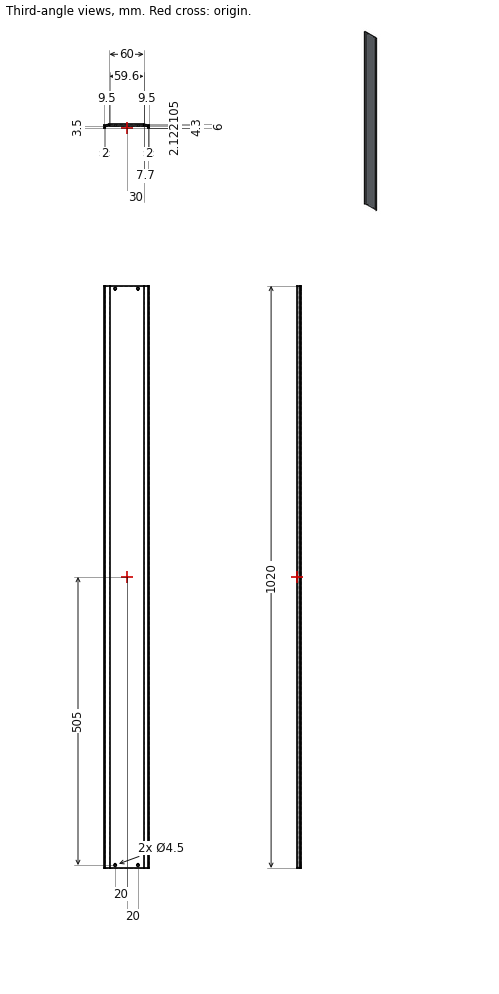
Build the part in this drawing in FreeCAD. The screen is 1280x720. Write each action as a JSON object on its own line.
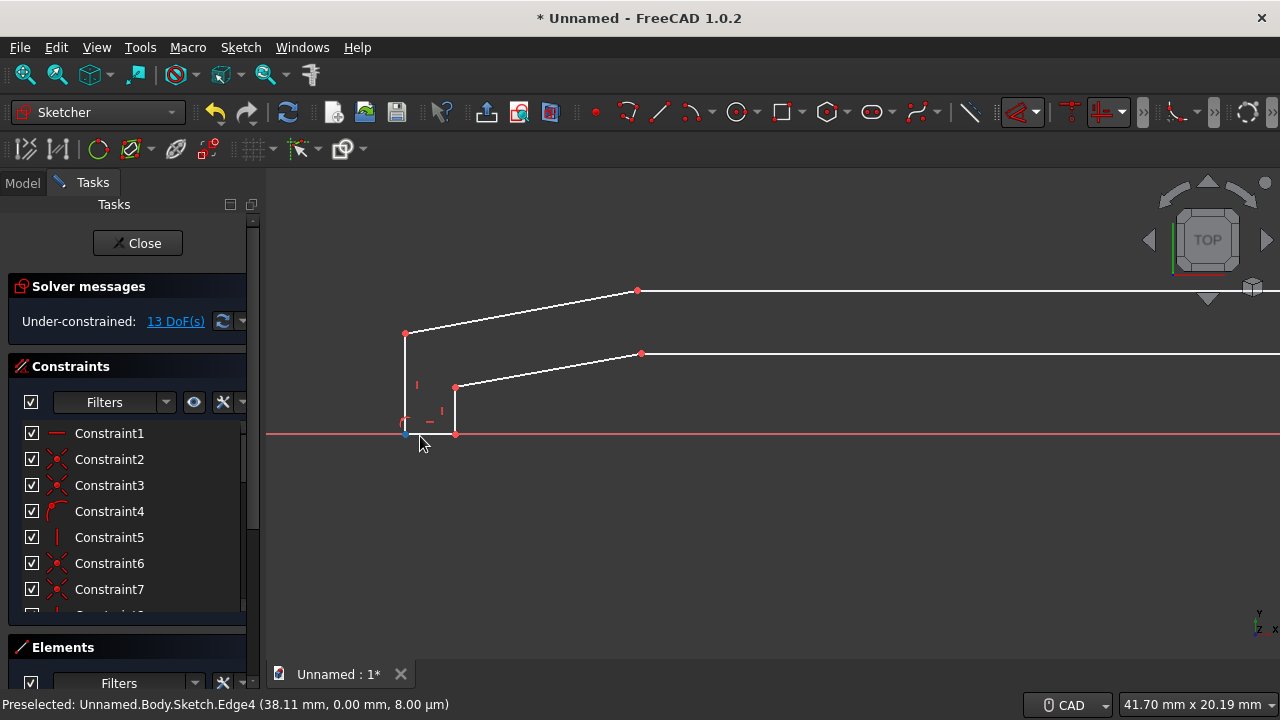
{"action": "left_click", "coordinate": [420, 434]}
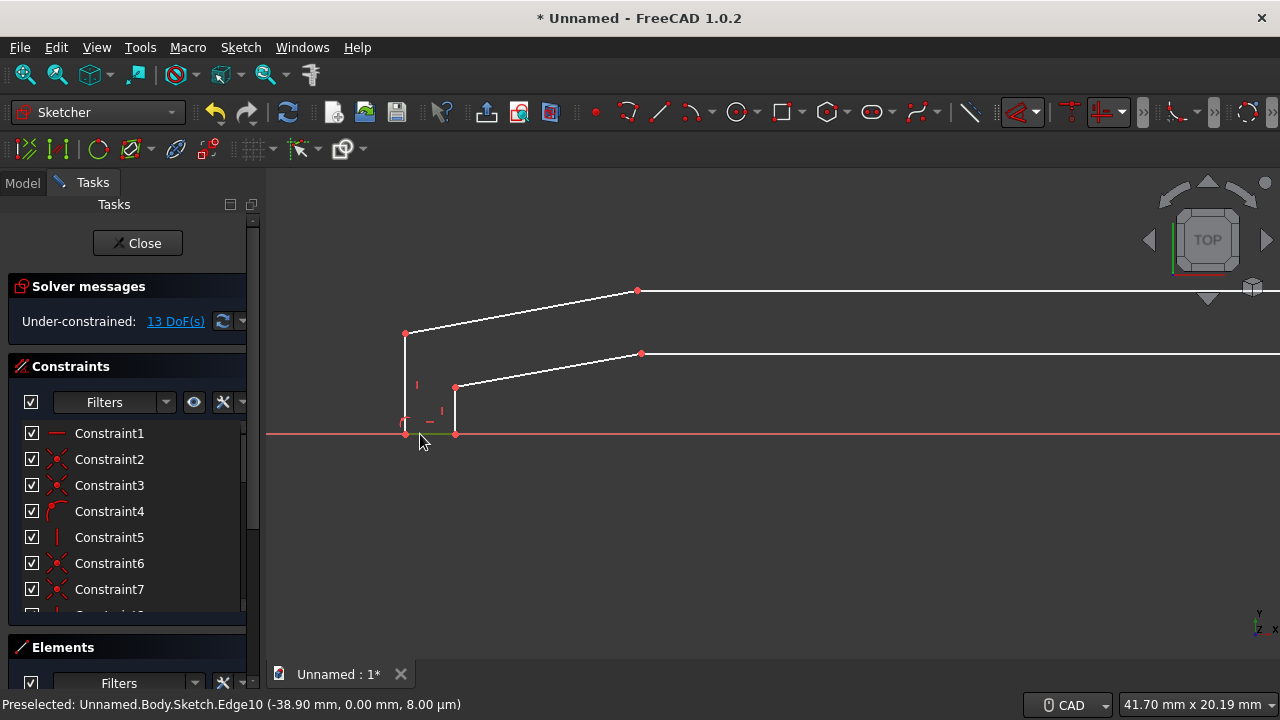
{"action": "key", "text": "l"}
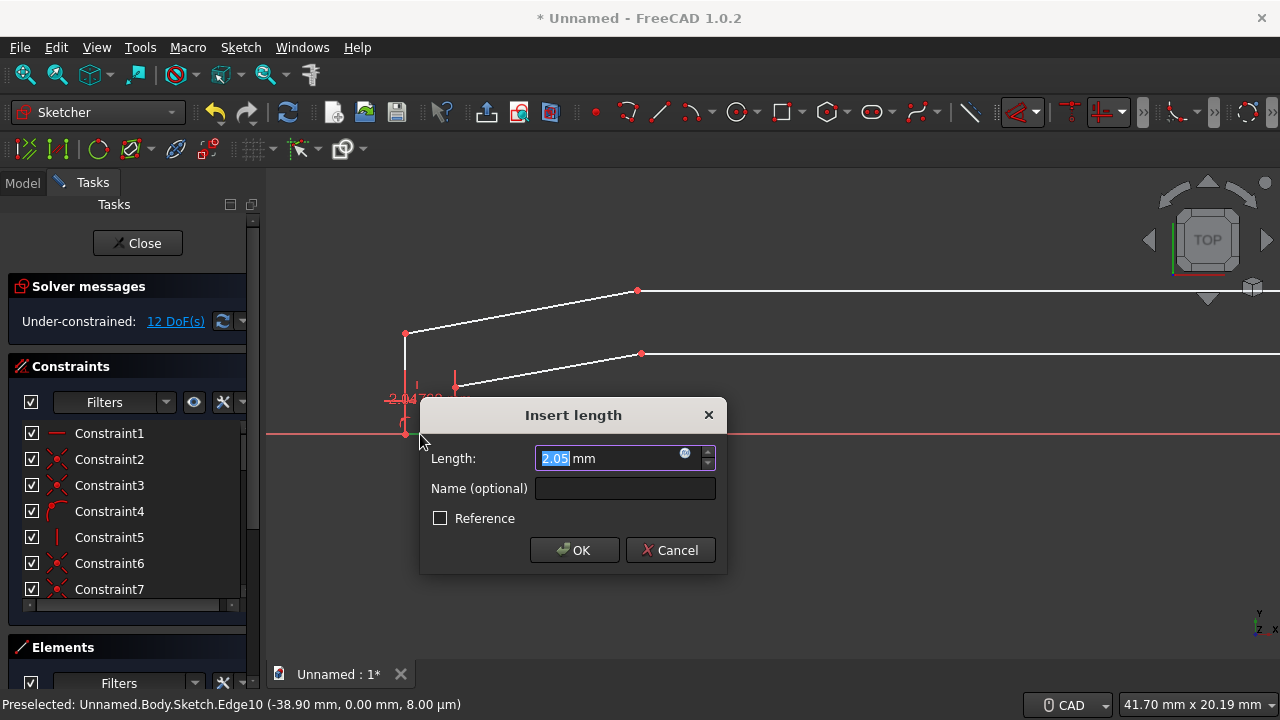
{"action": "type", "text": "2"}
{"action": "key", "text": "Return"}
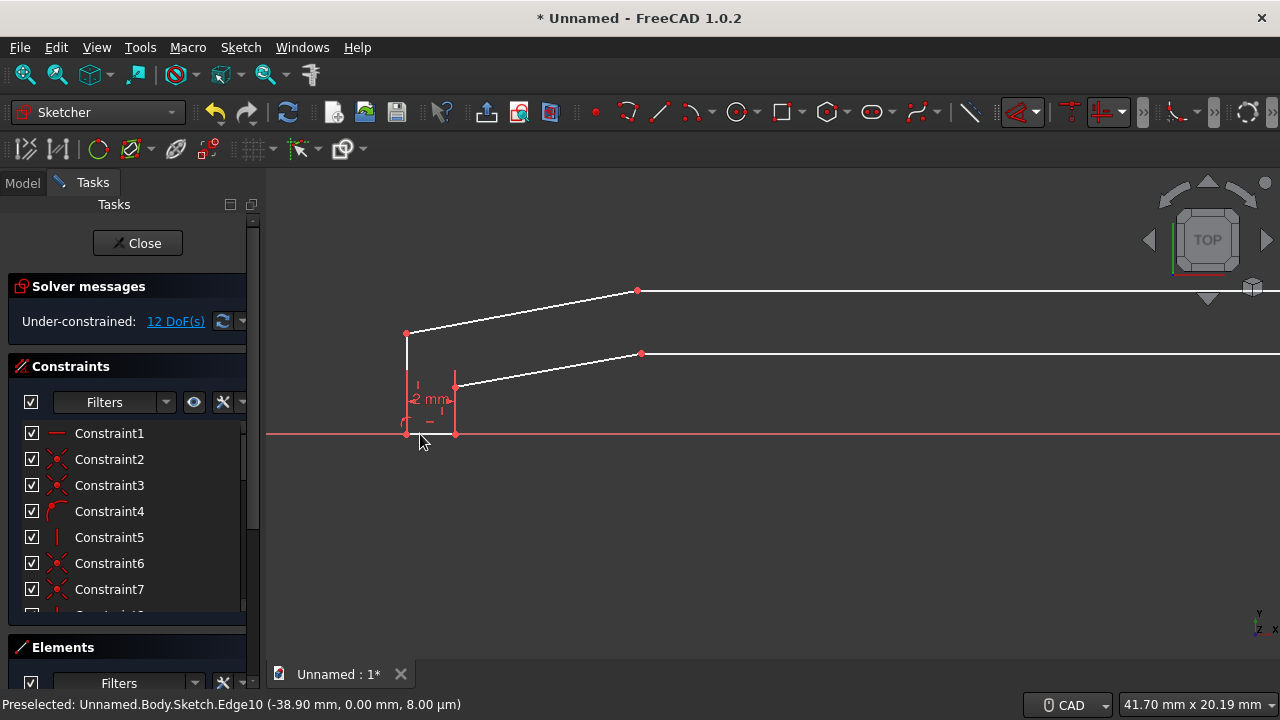
{"action": "left_click", "coordinate": [1075, 291]}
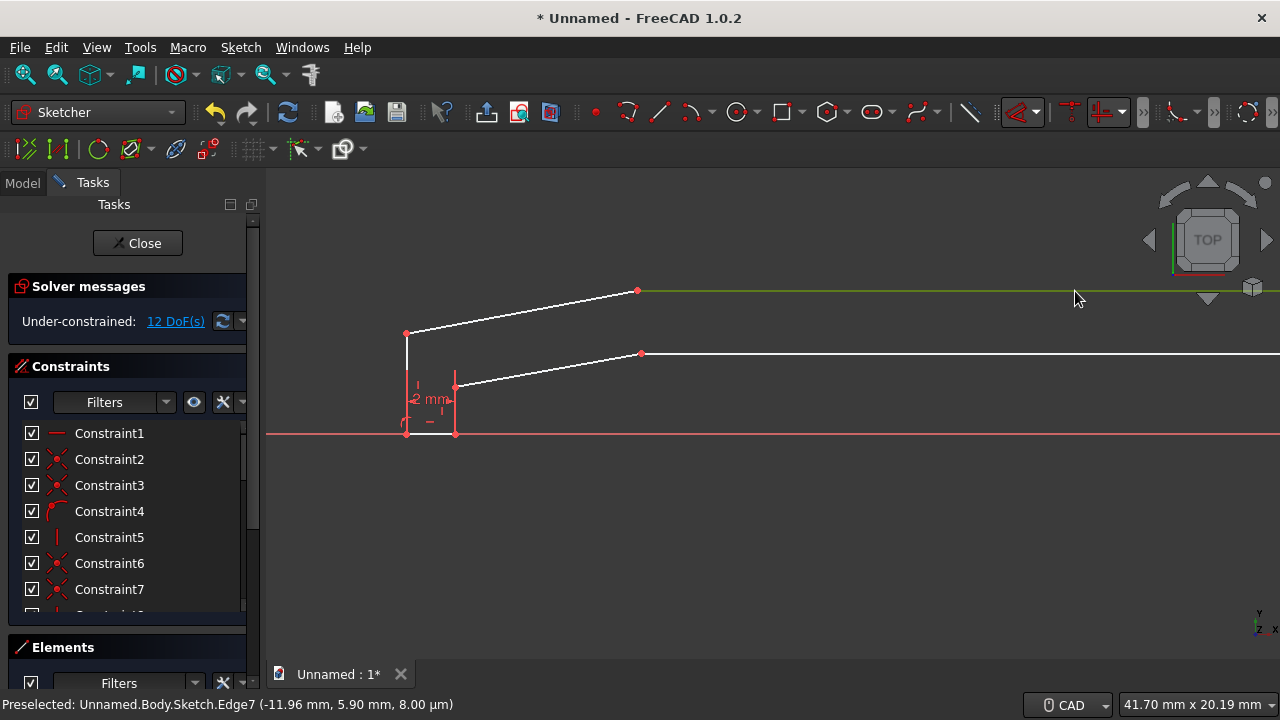
{"action": "left_click", "coordinate": [1038, 112]}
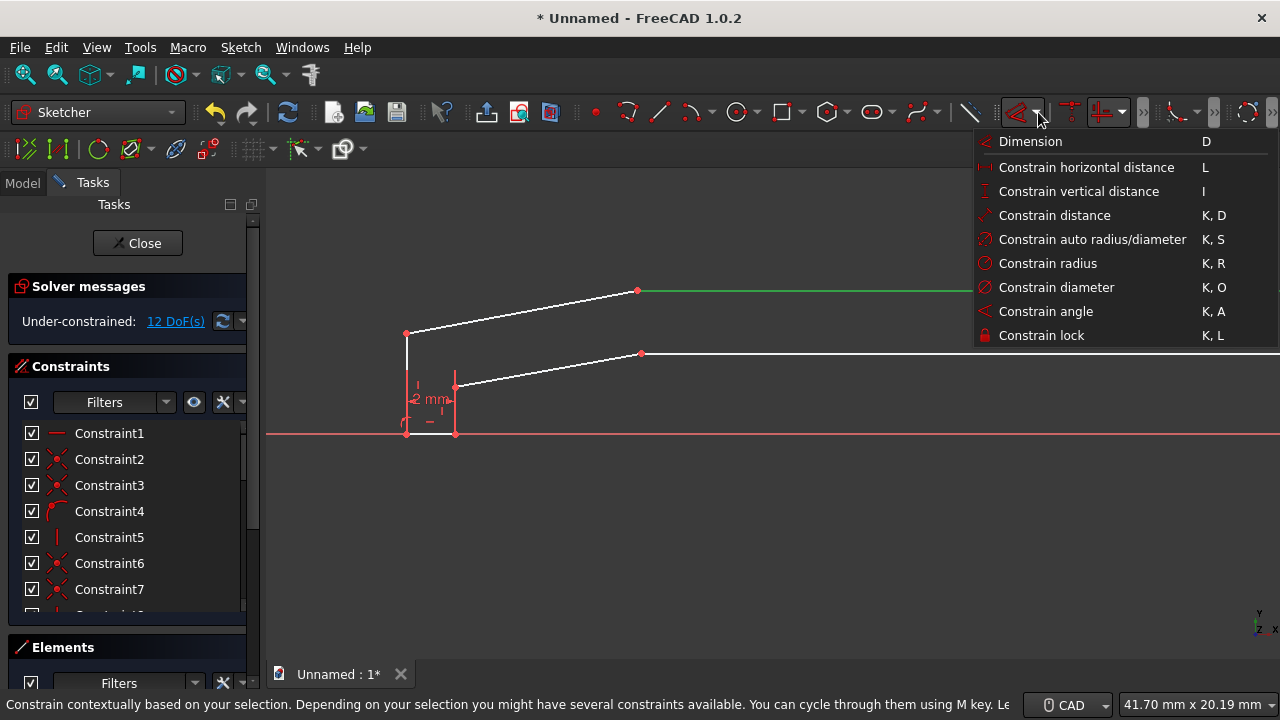
{"action": "left_click", "coordinate": [1126, 167]}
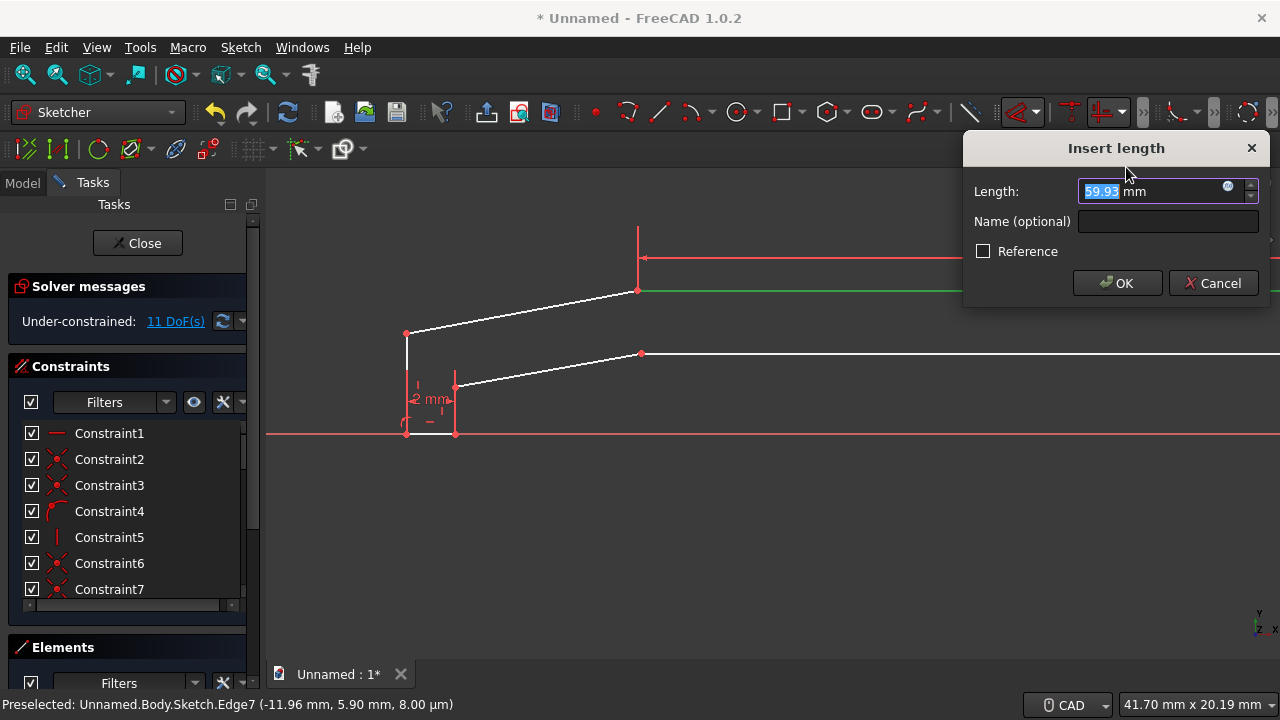
{"action": "type", "text": "60"}
{"action": "key", "text": "Return"}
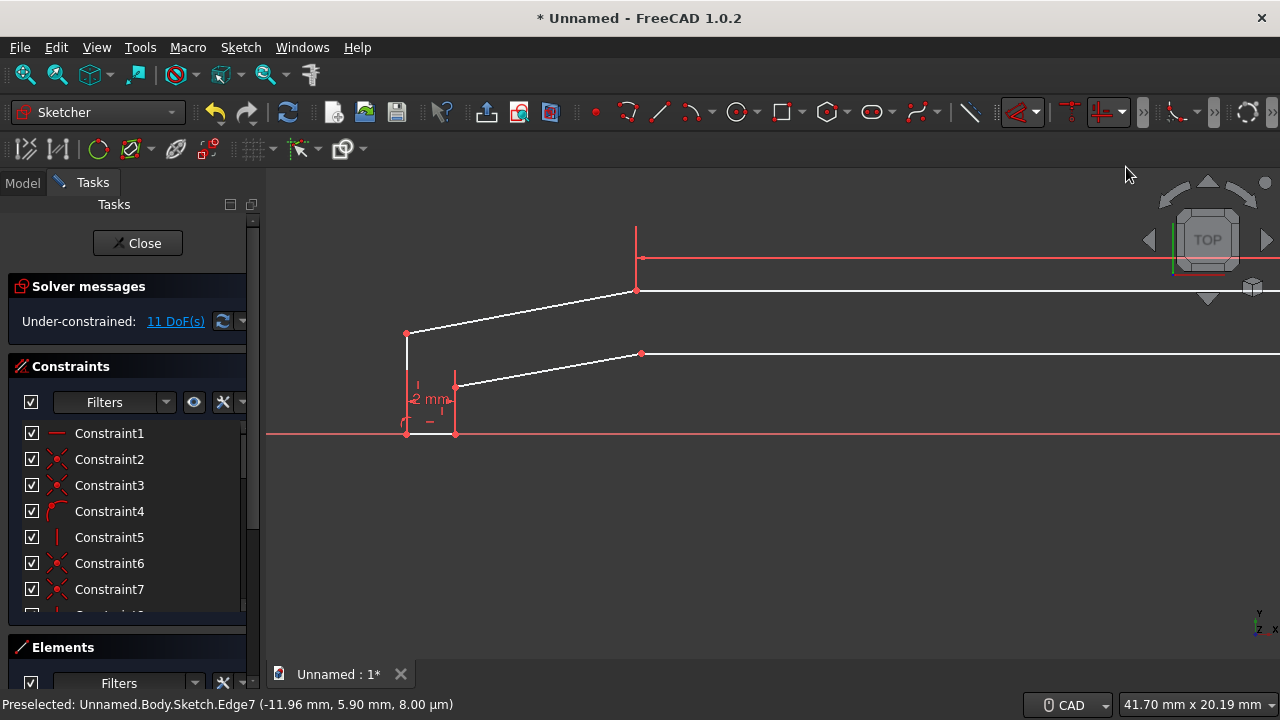
{"action": "scroll", "coordinate": [419, 436], "scroll_direction": "down", "scroll_amount": 6}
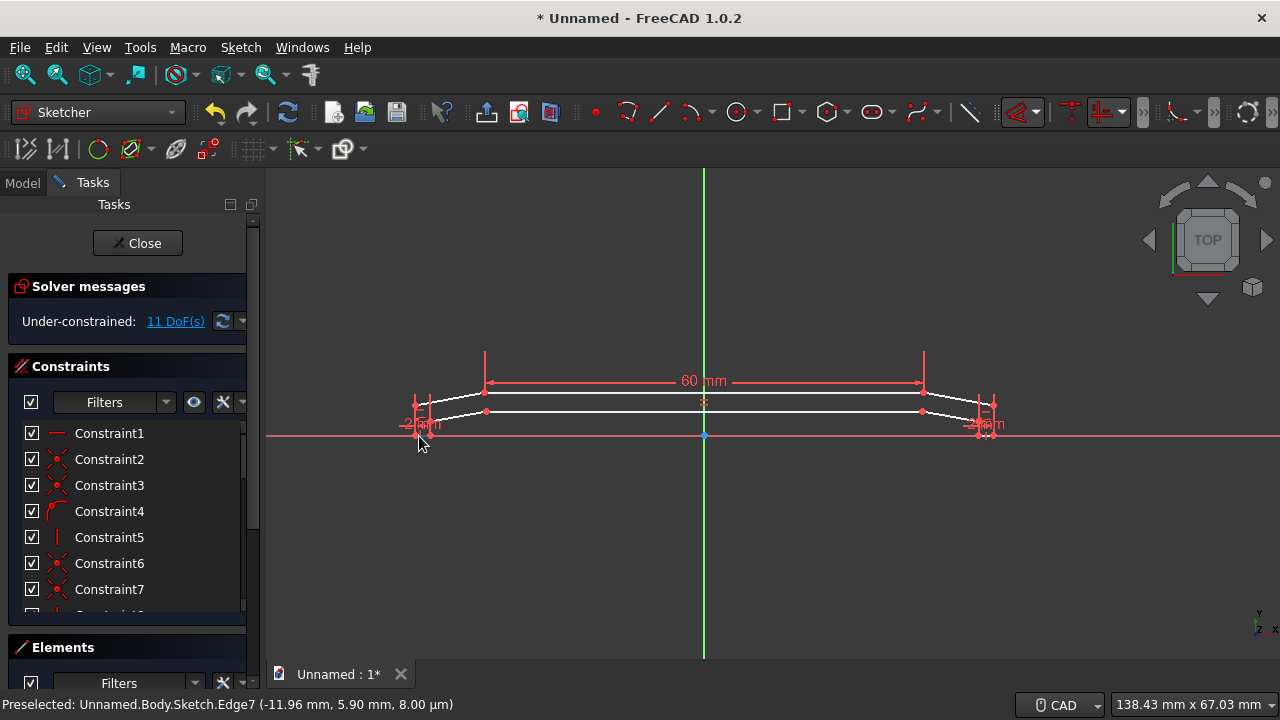
{"action": "left_click", "coordinate": [924, 393]}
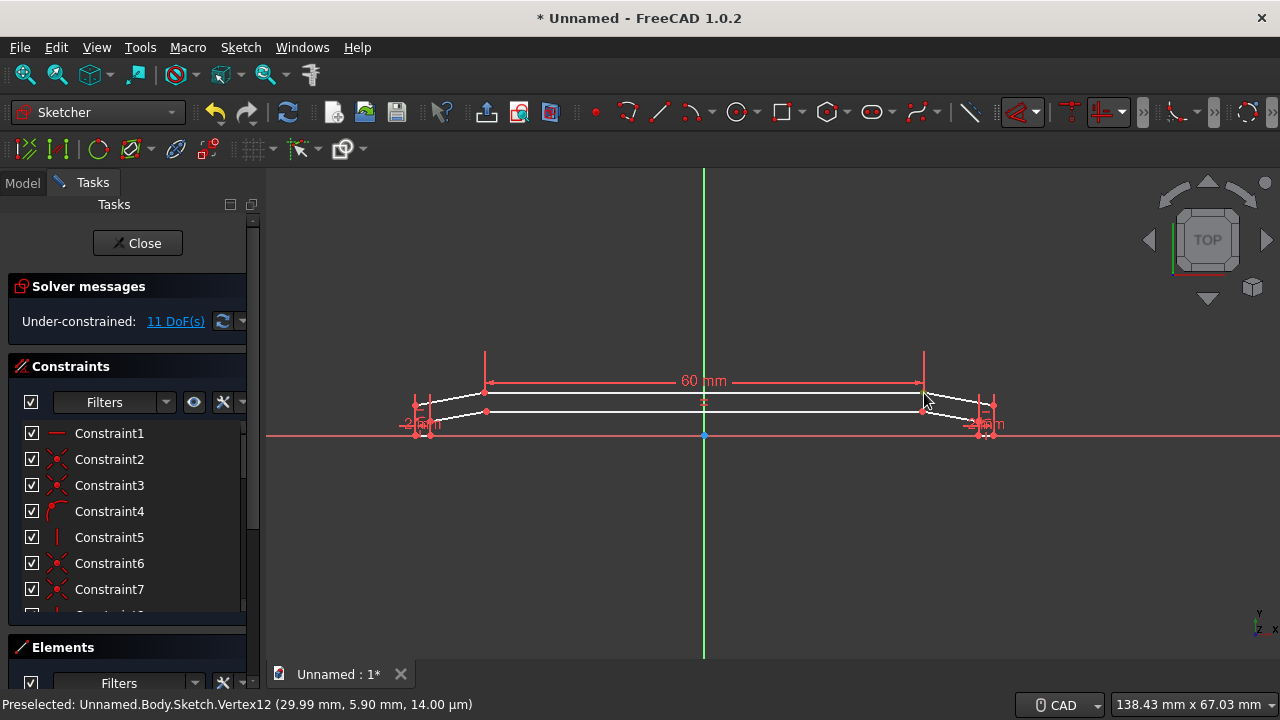
{"action": "left_click", "coordinate": [1038, 112]}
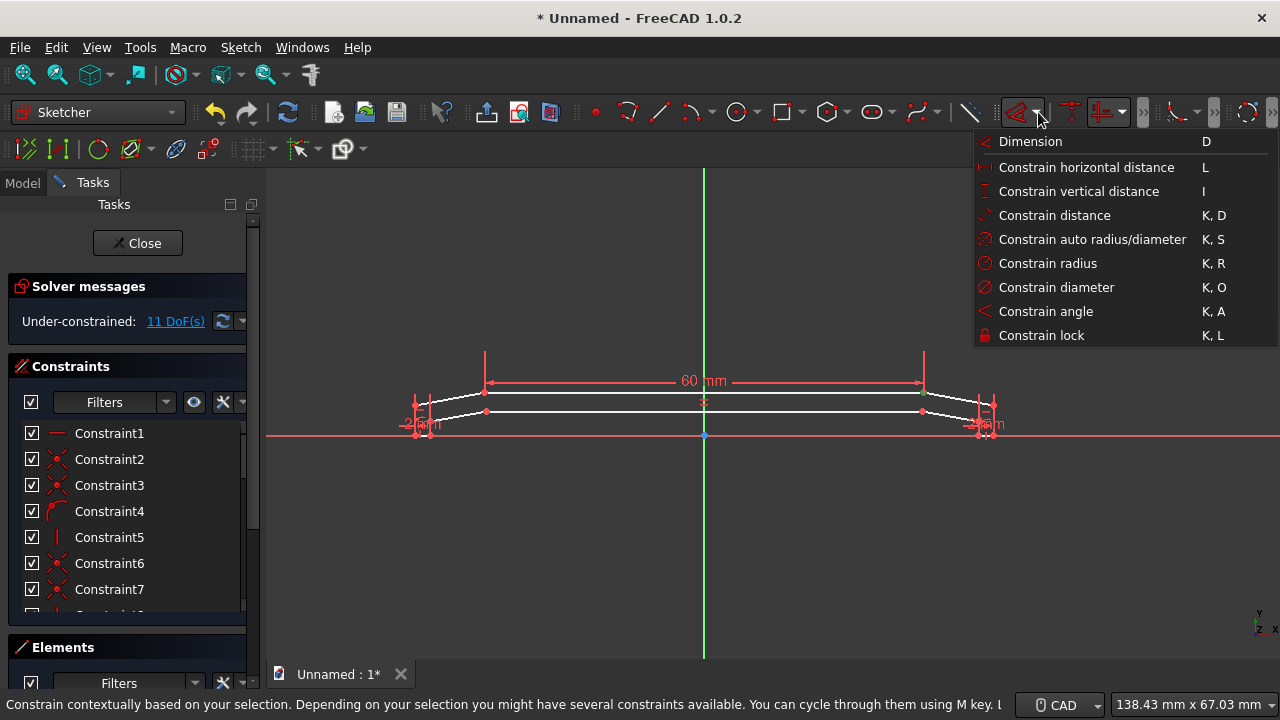
{"action": "left_click", "coordinate": [1126, 191]}